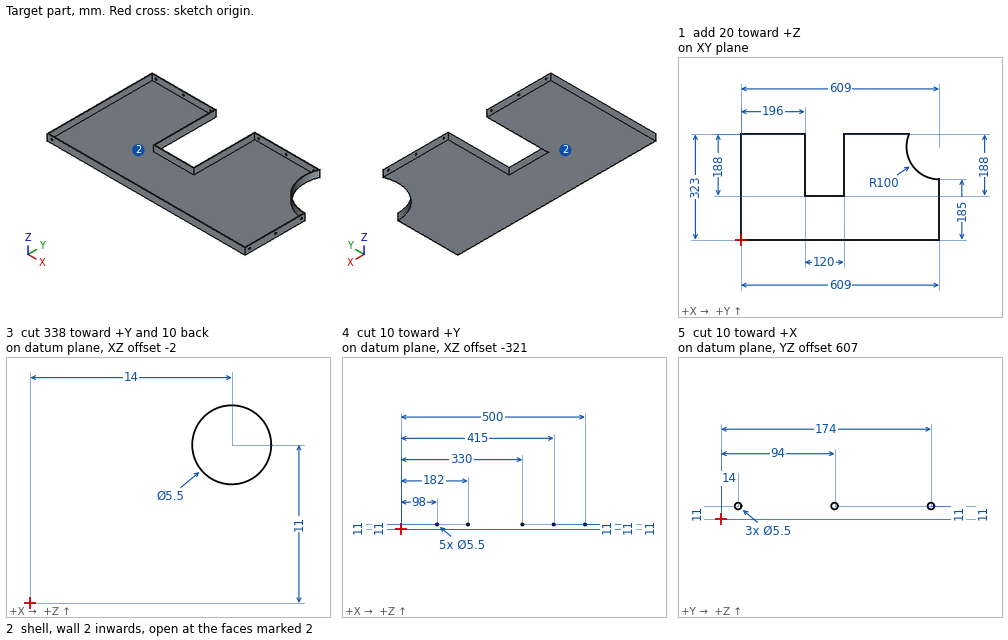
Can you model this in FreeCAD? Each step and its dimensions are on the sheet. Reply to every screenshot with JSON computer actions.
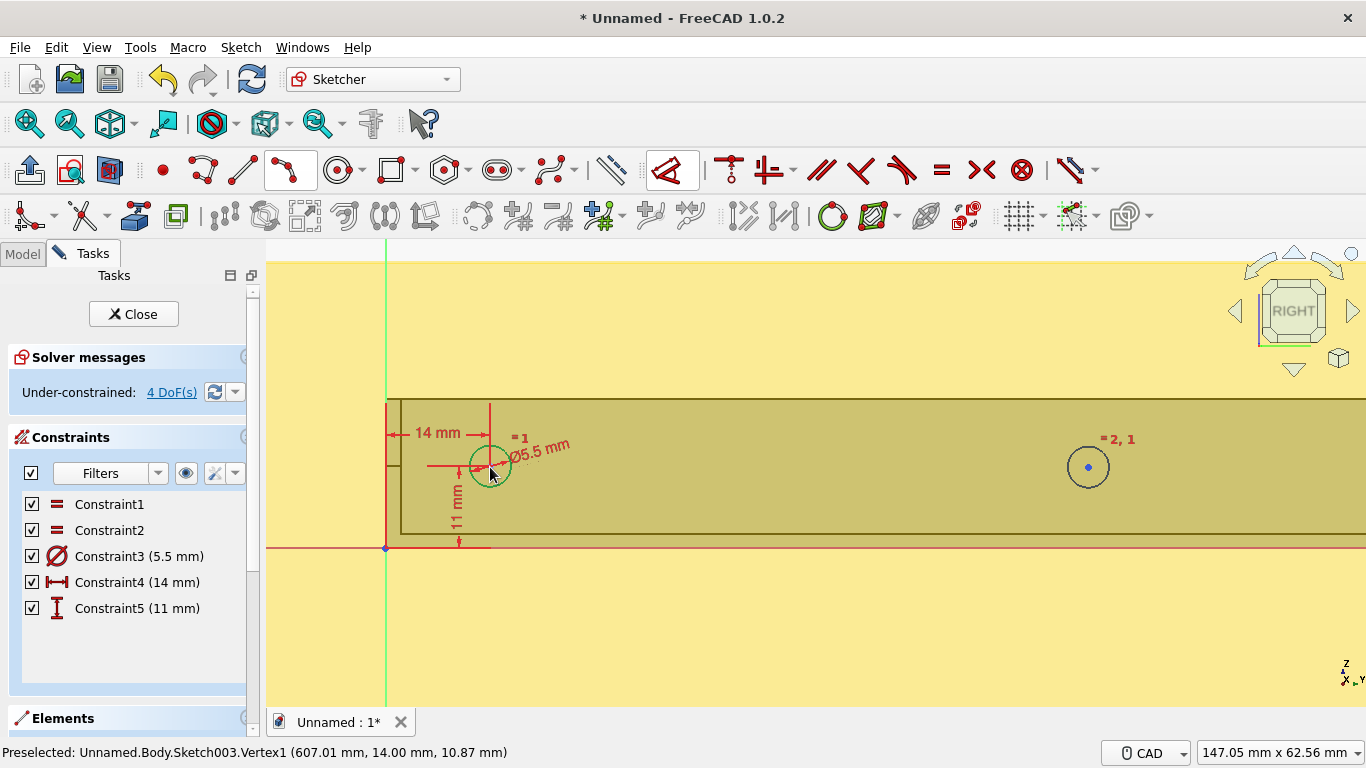
{"action": "left_click", "coordinate": [1088, 467]}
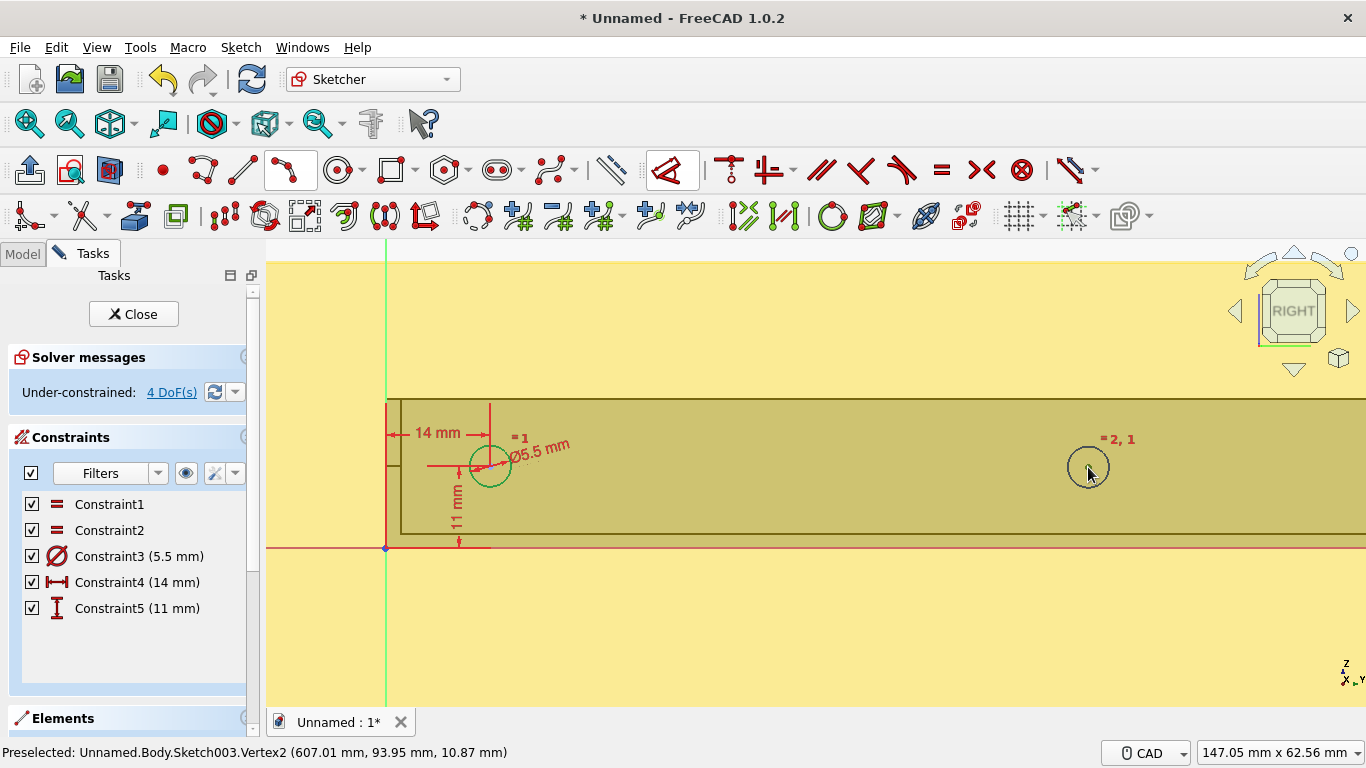
{"action": "key", "text": "l"}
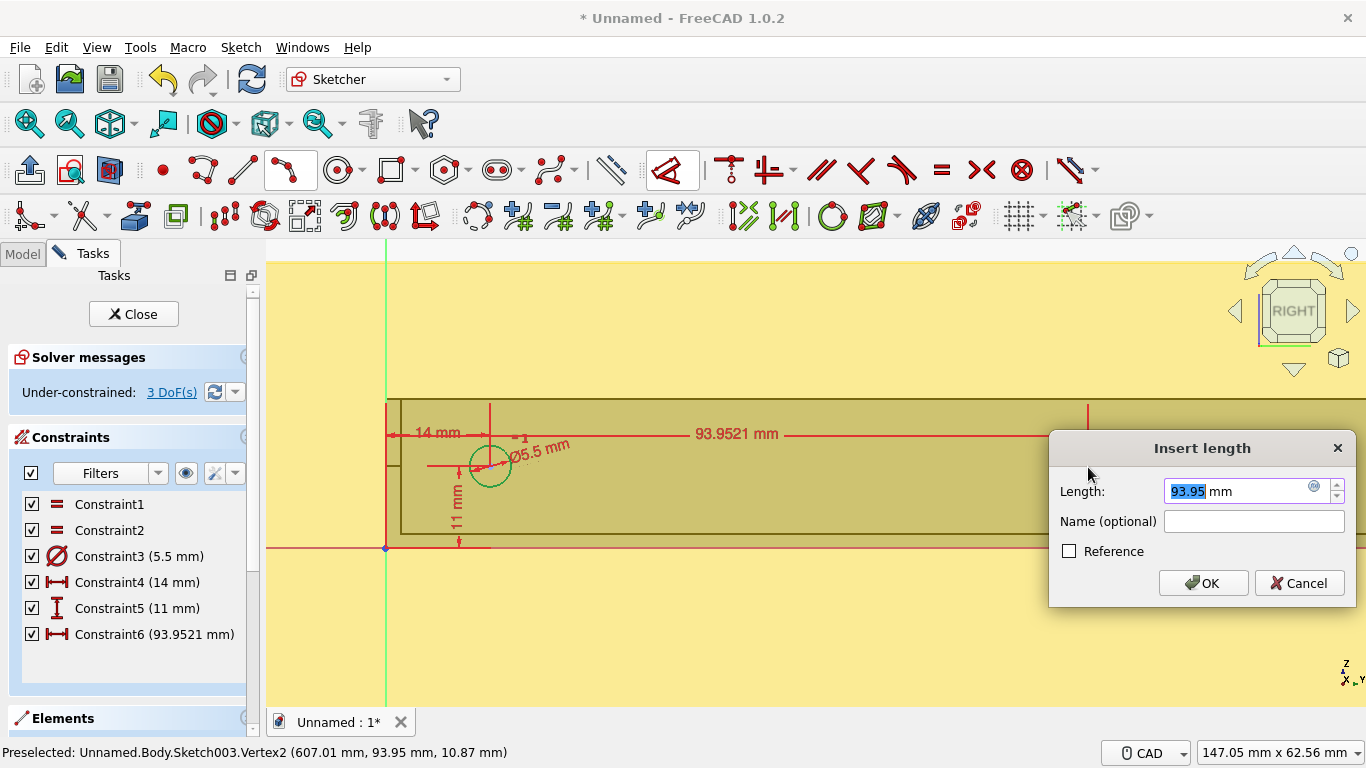
{"action": "type", "text": "94"}
{"action": "key", "text": "Return"}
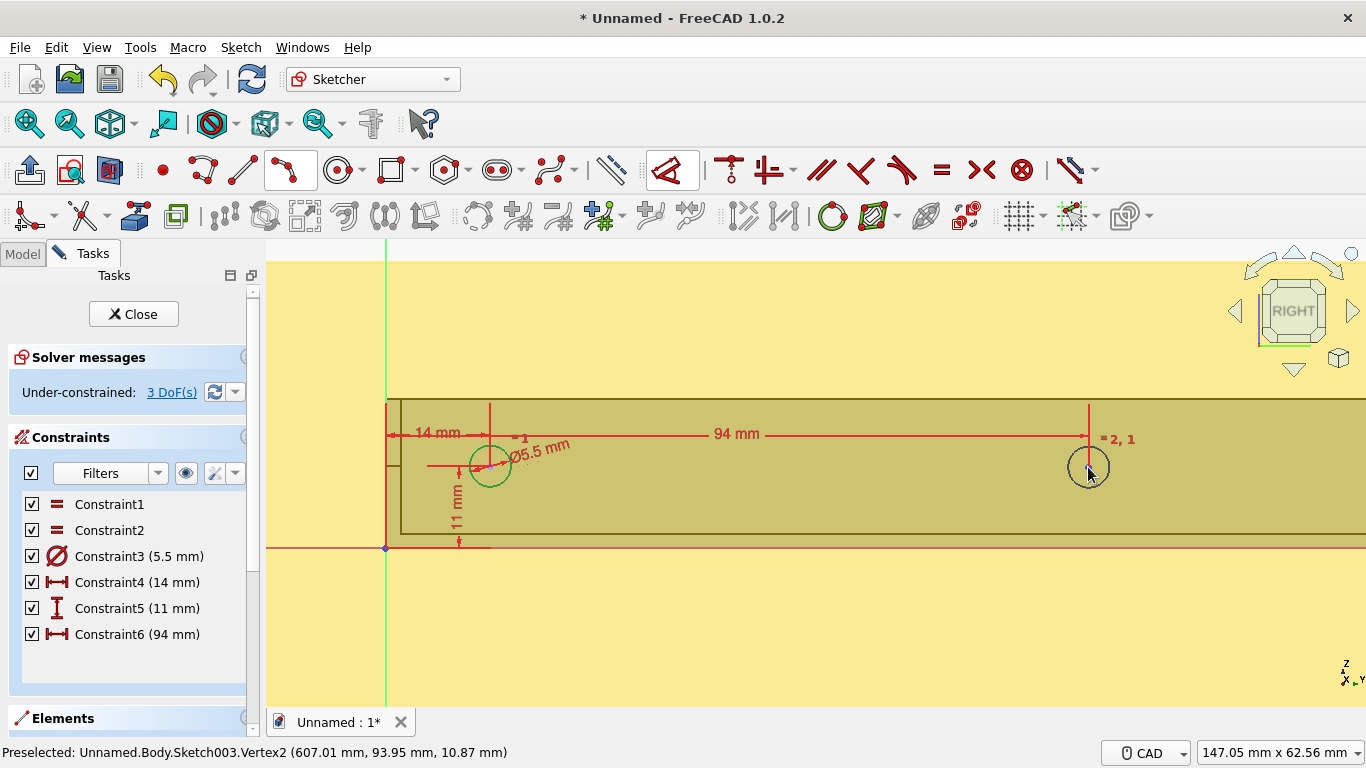
{"action": "left_click", "coordinate": [1089, 467]}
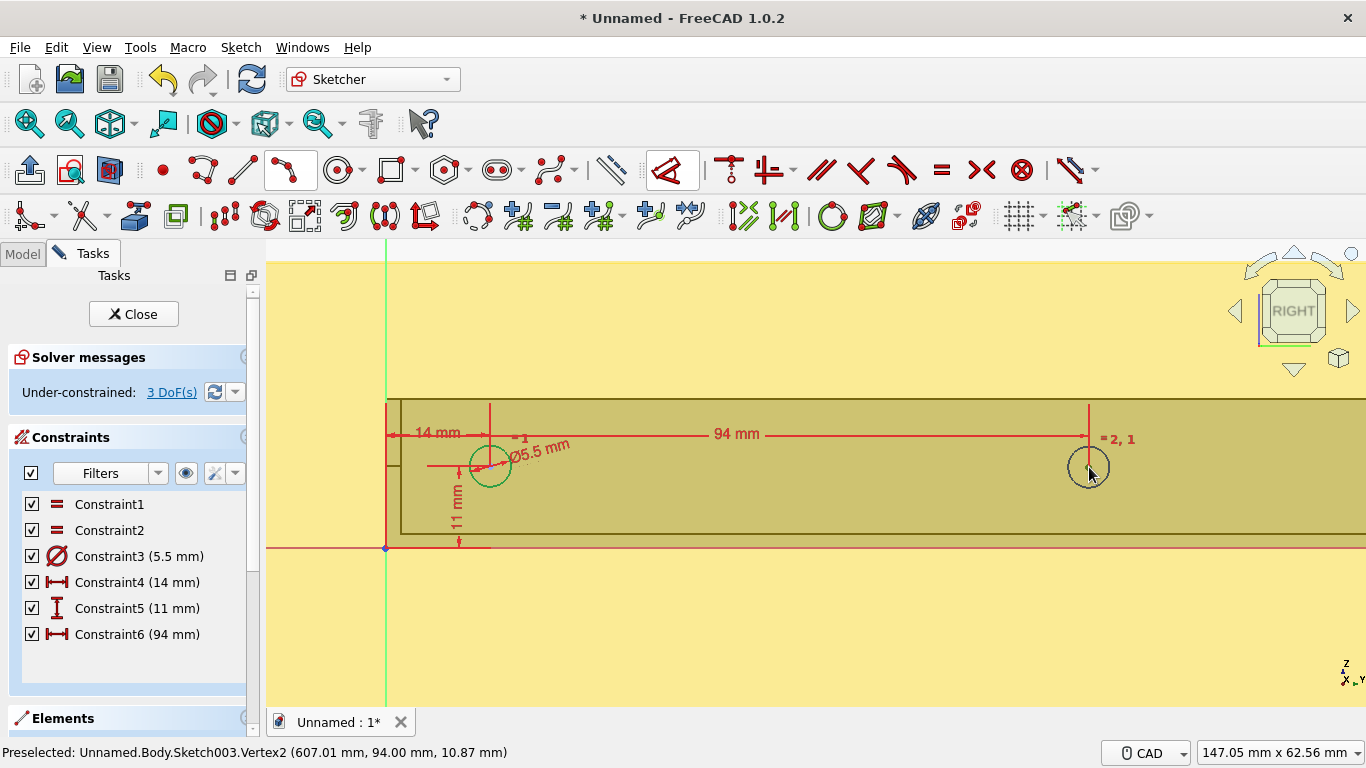
{"action": "key", "text": "i"}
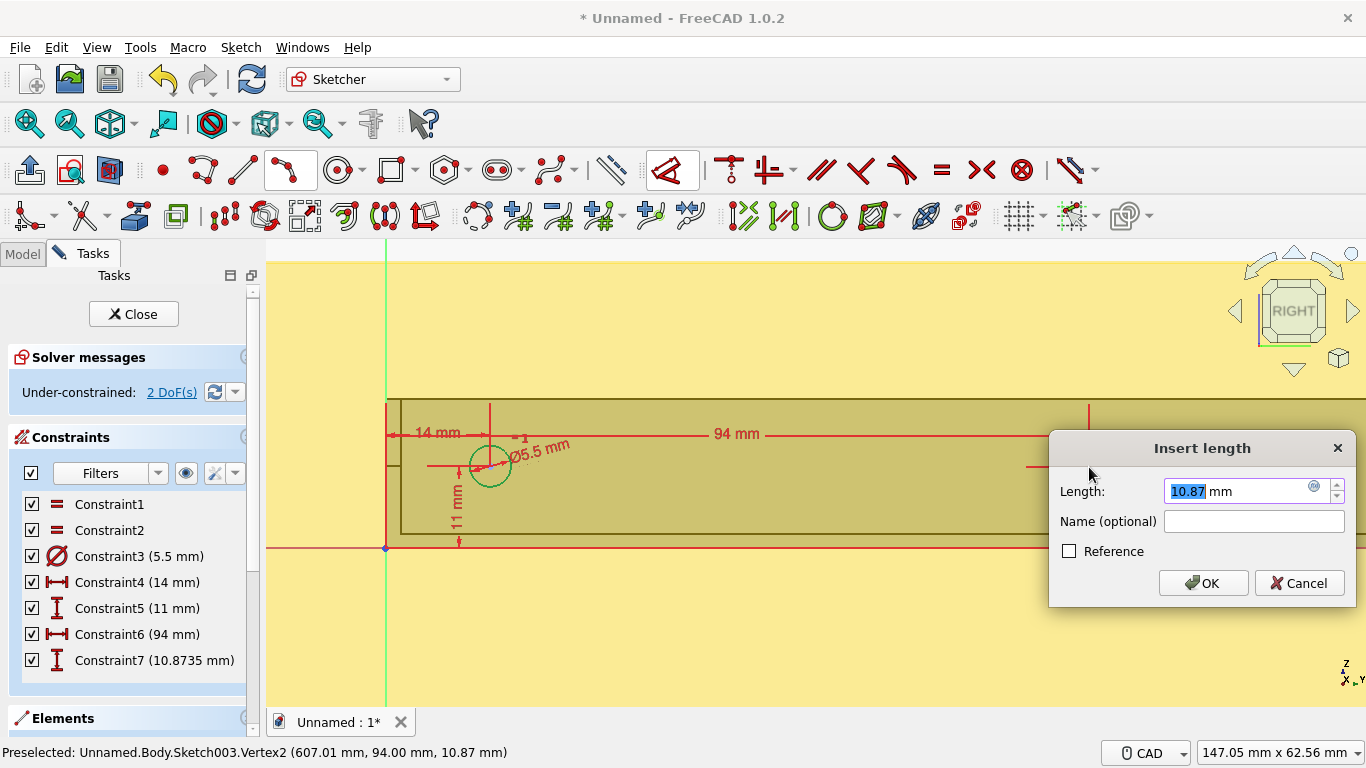
{"action": "type", "text": "11"}
{"action": "key", "text": "Return"}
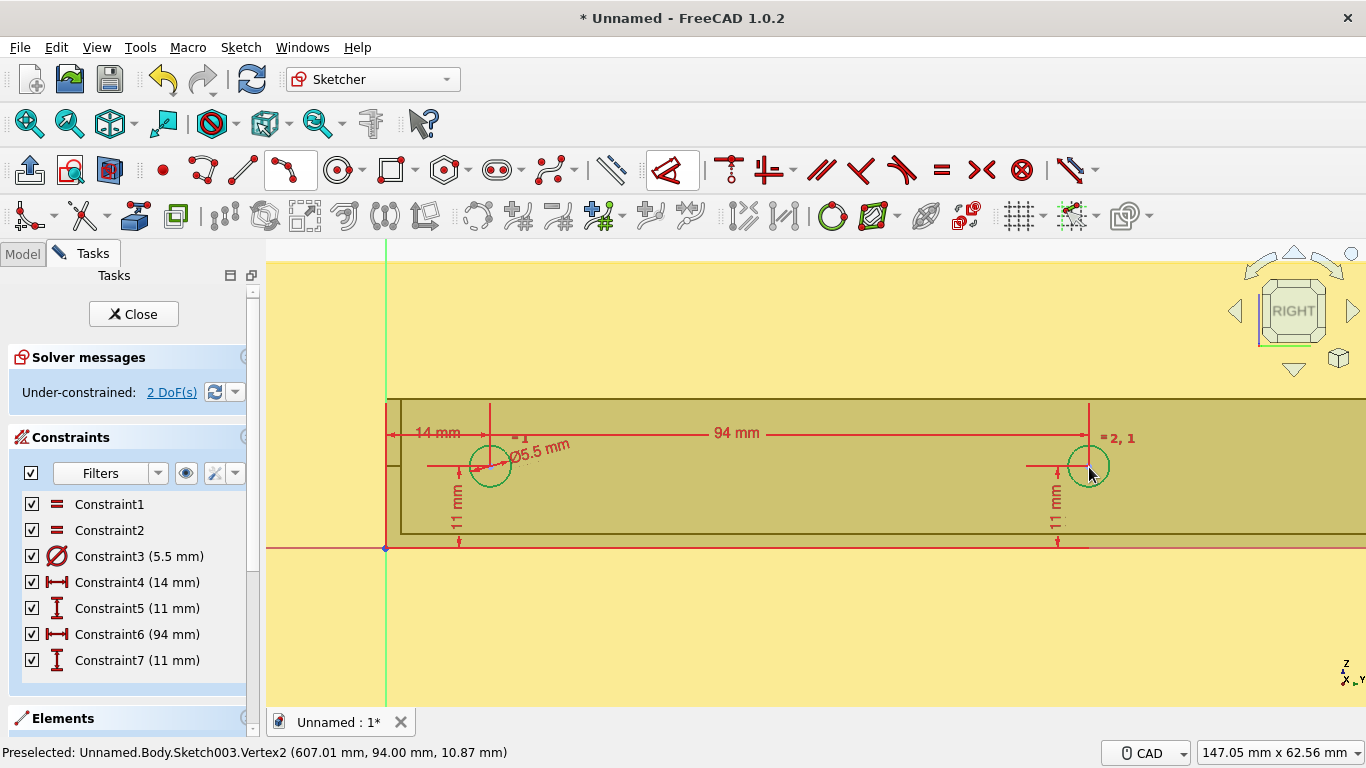
{"action": "scroll", "coordinate": [503, 453], "scroll_direction": "down", "scroll_amount": 4}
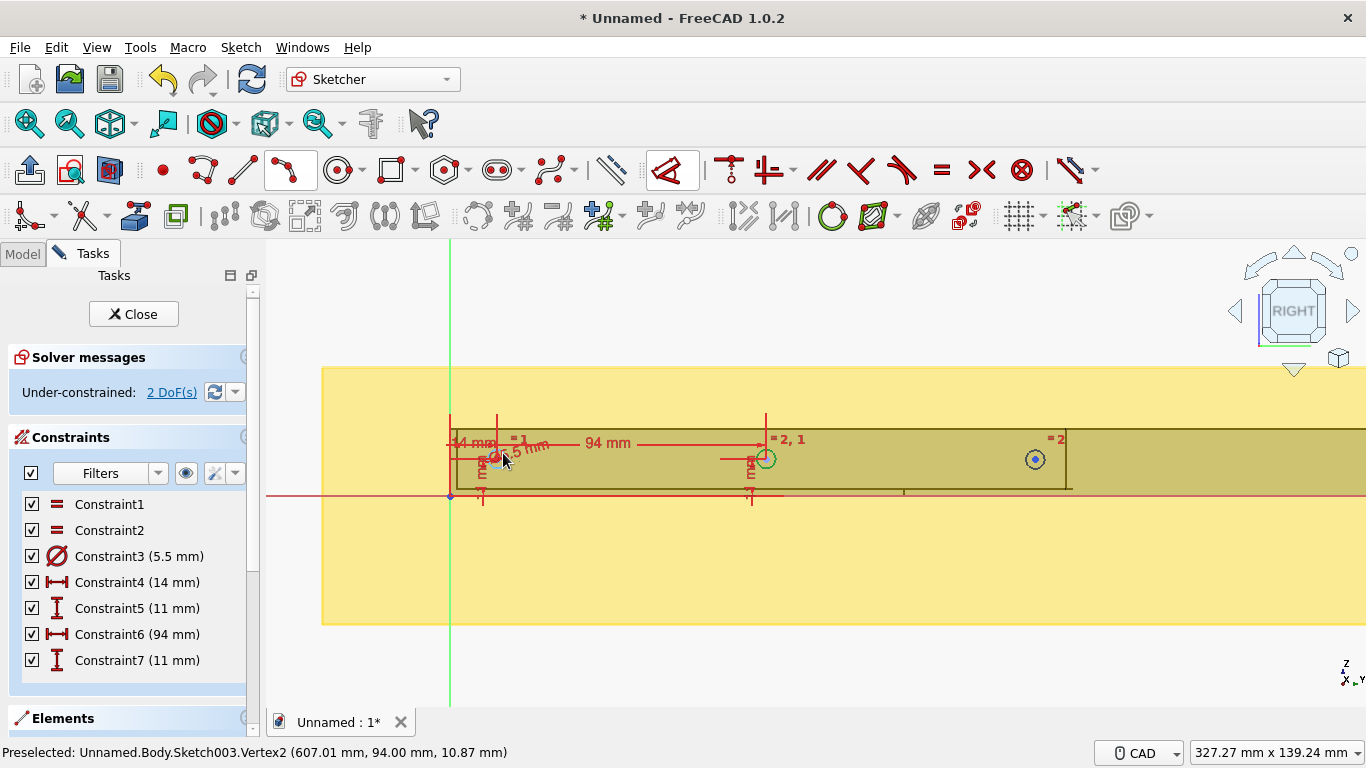
{"action": "left_click", "coordinate": [1035, 460]}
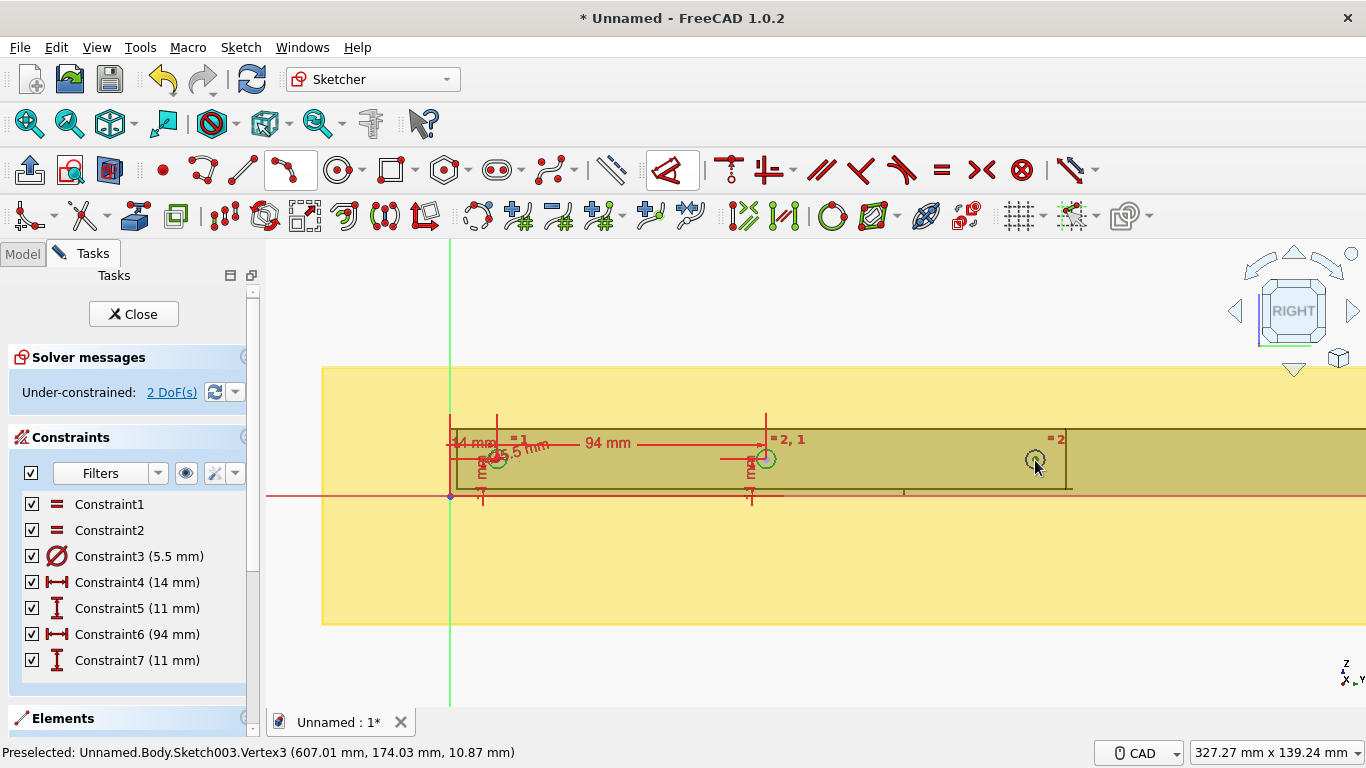
{"action": "key", "text": "i"}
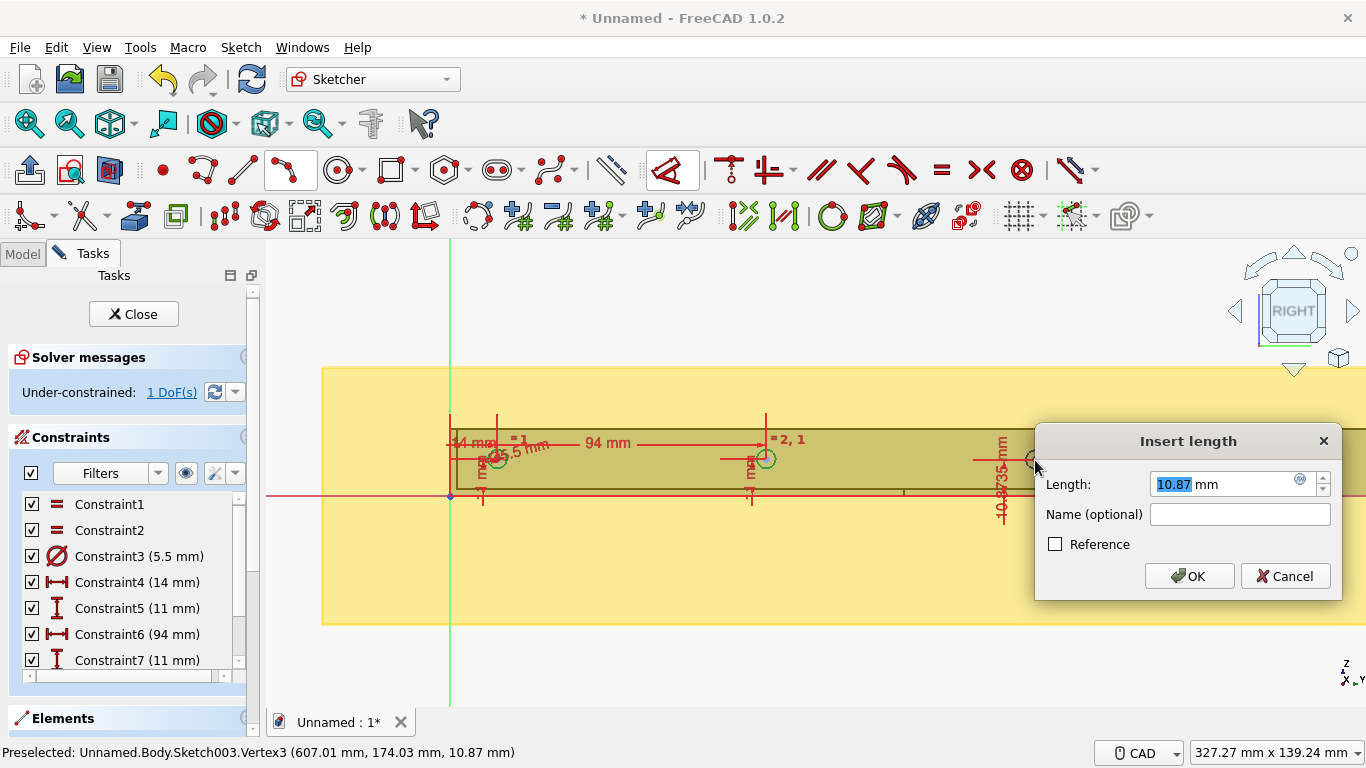
{"action": "type", "text": "11"}
{"action": "key", "text": "Return"}